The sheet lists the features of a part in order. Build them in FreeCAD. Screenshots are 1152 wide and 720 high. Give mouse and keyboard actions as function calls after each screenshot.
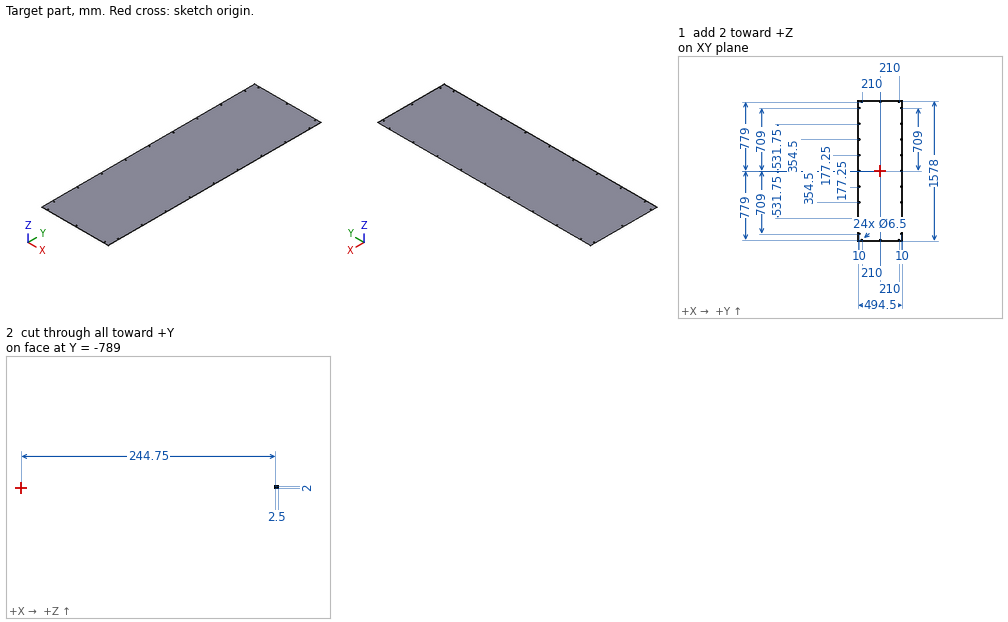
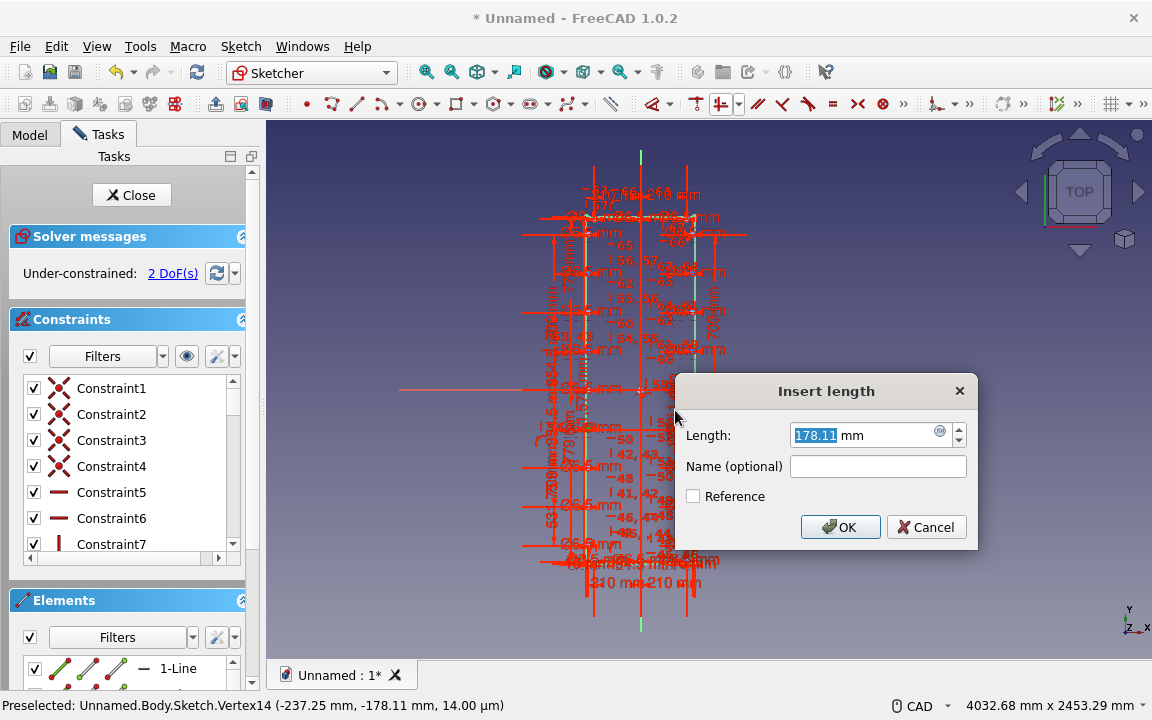
text(177.25)
key(Return)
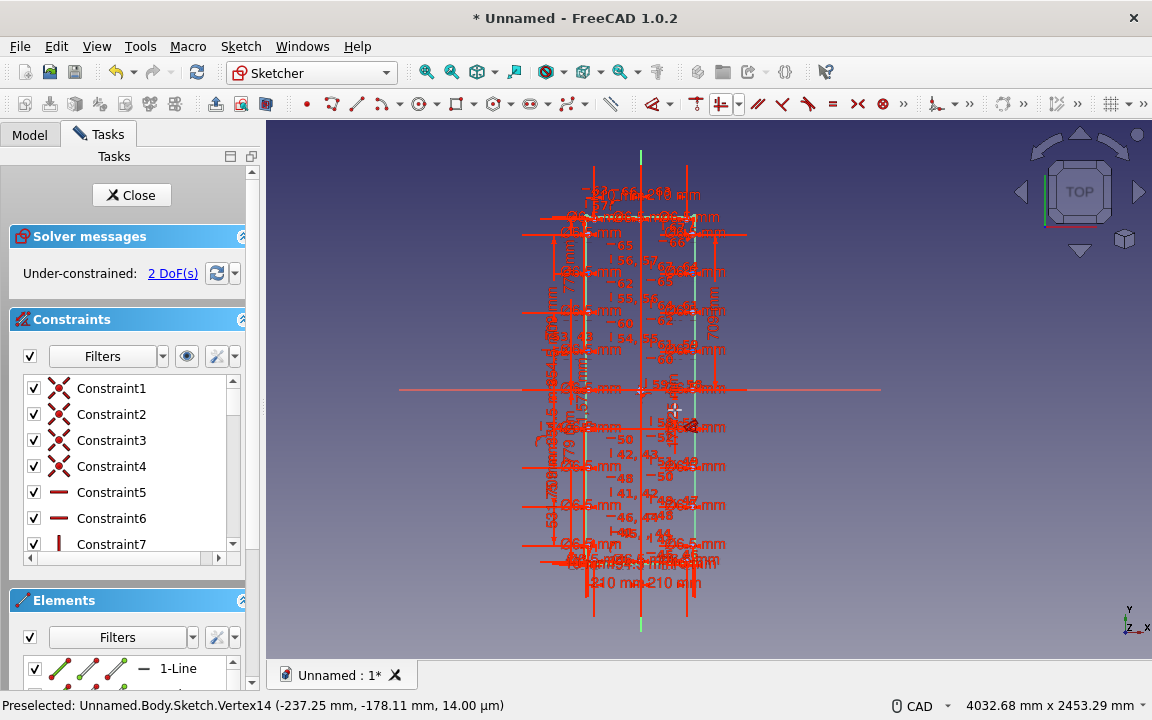
click(588, 352)
click(675, 371)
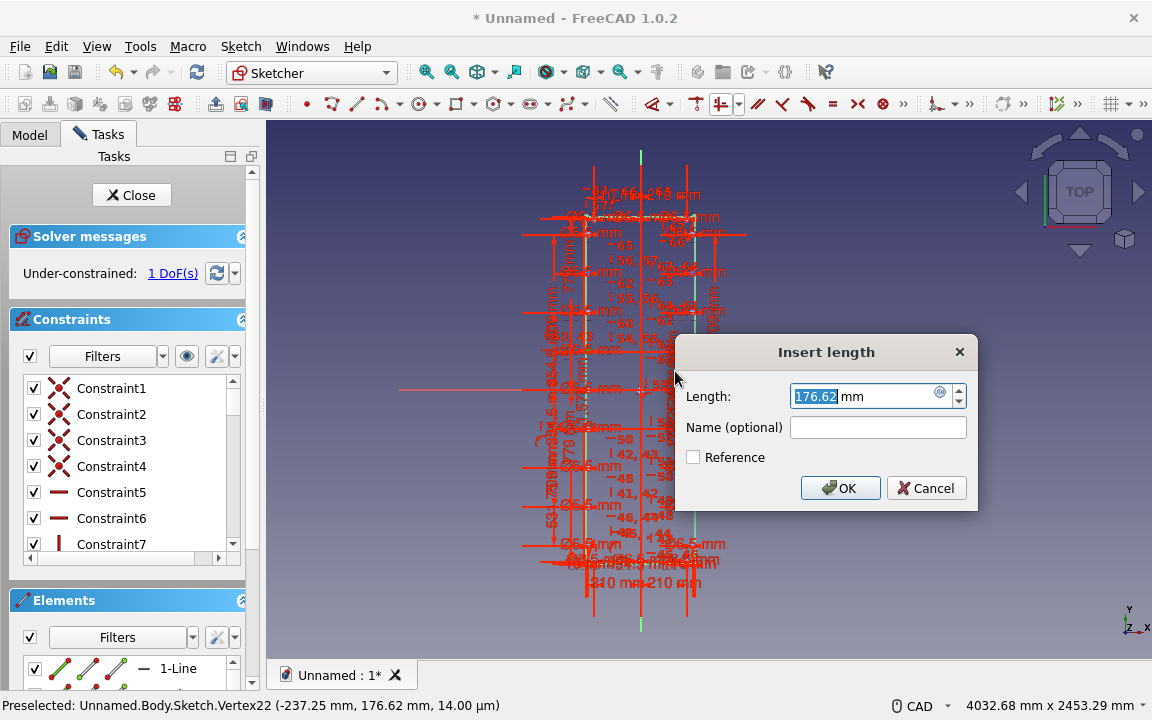
text(177.25)
key(Return)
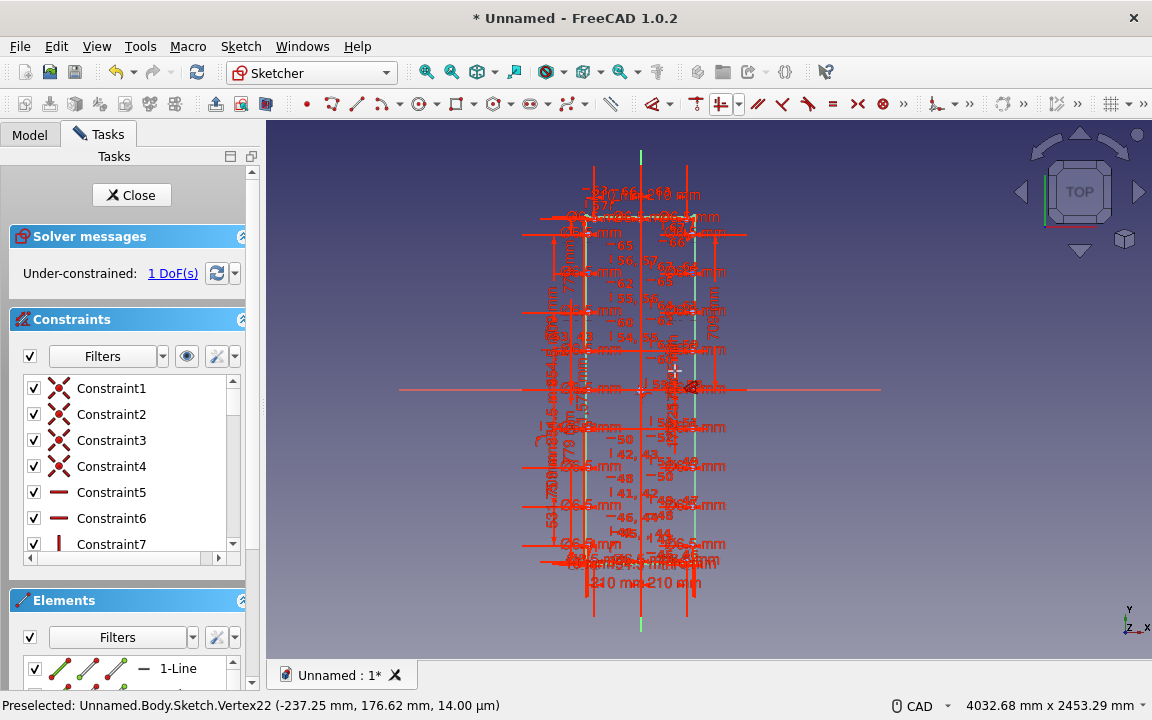
click(588, 274)
click(554, 291)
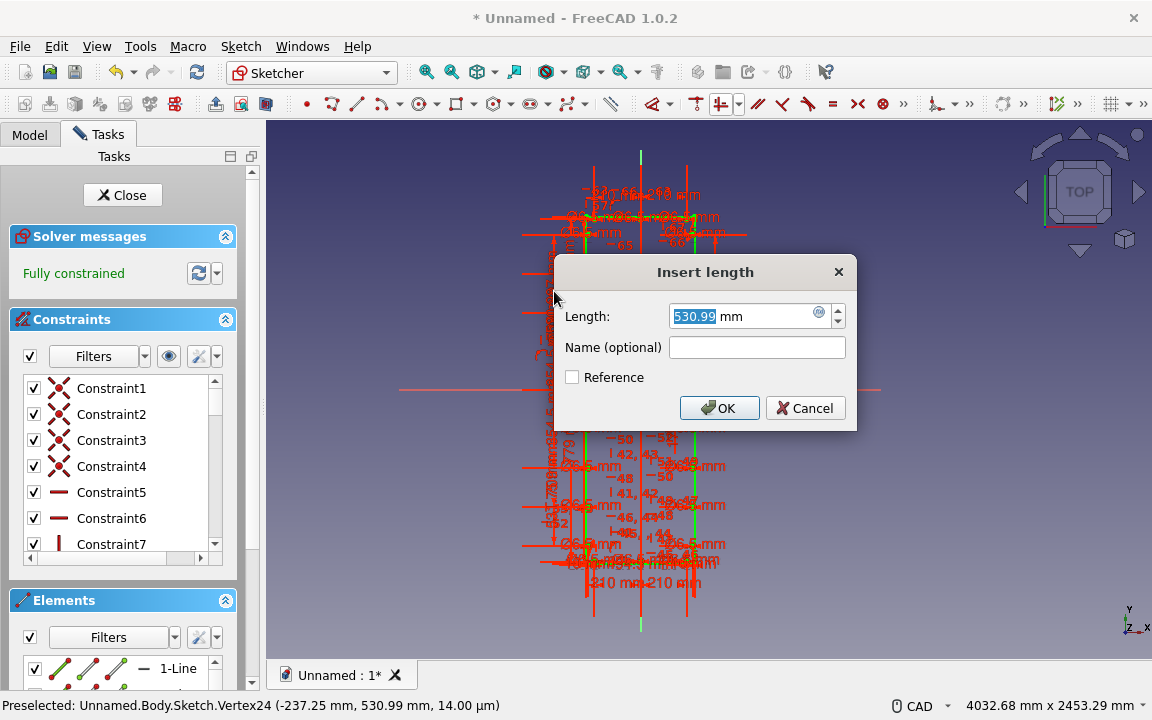
text(531.75)
key(Return)
key(Escape)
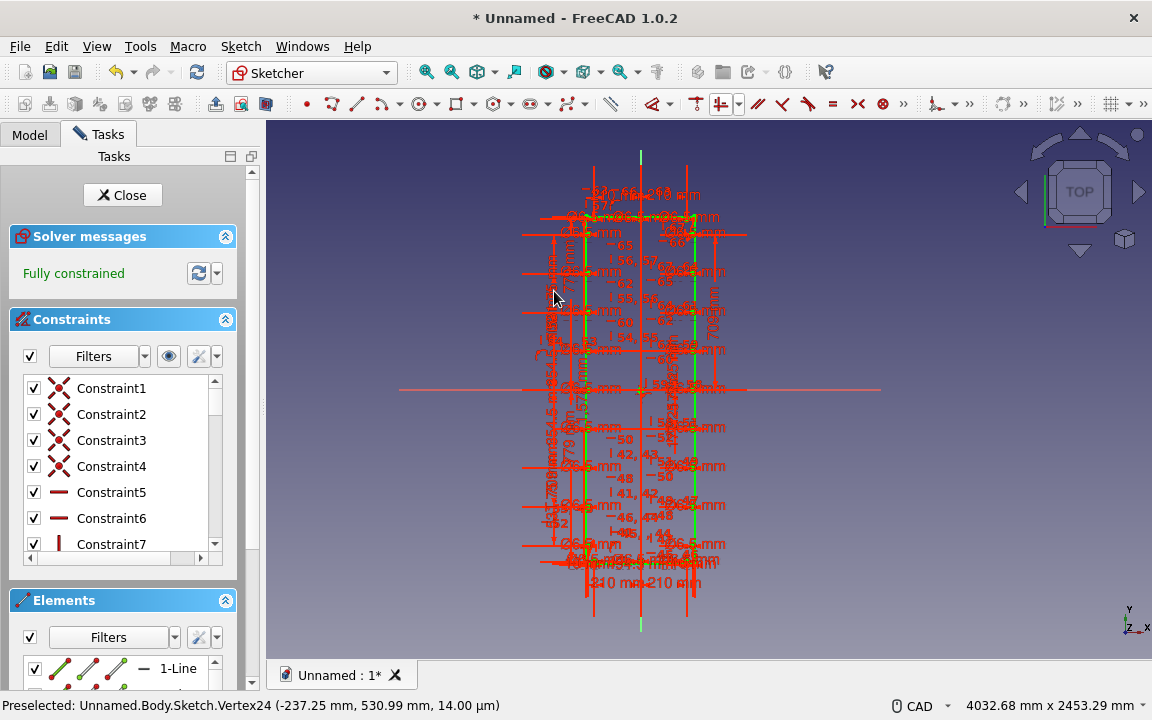
click(123, 195)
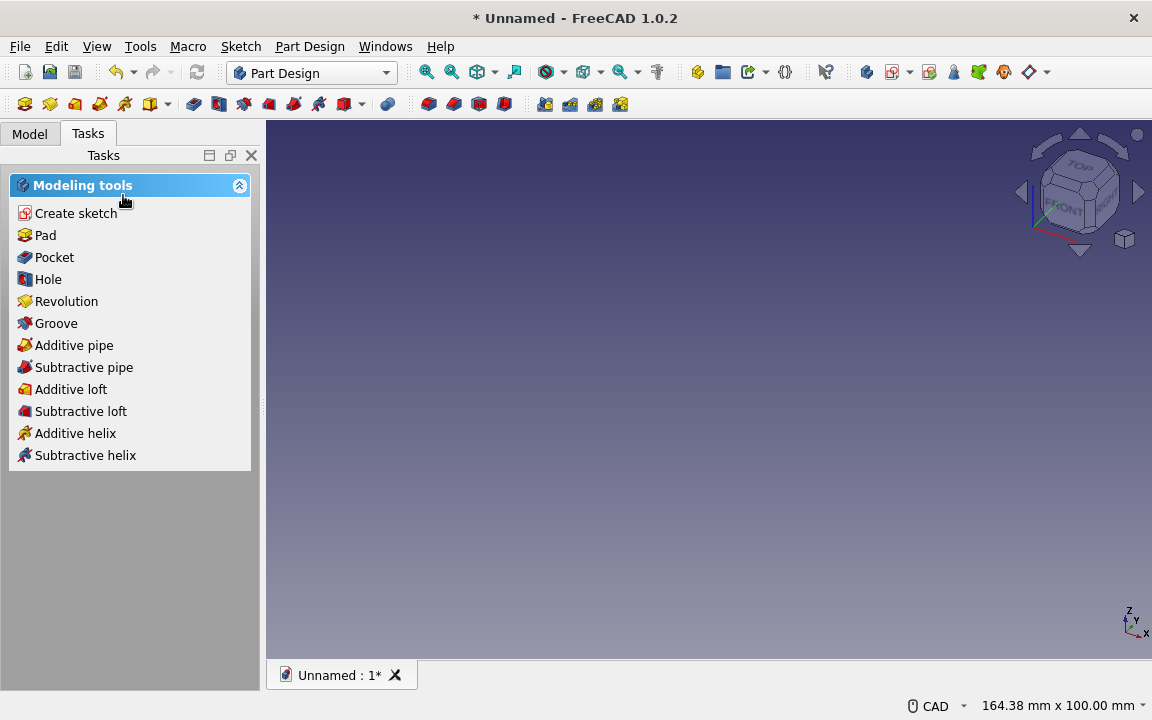
click(25, 104)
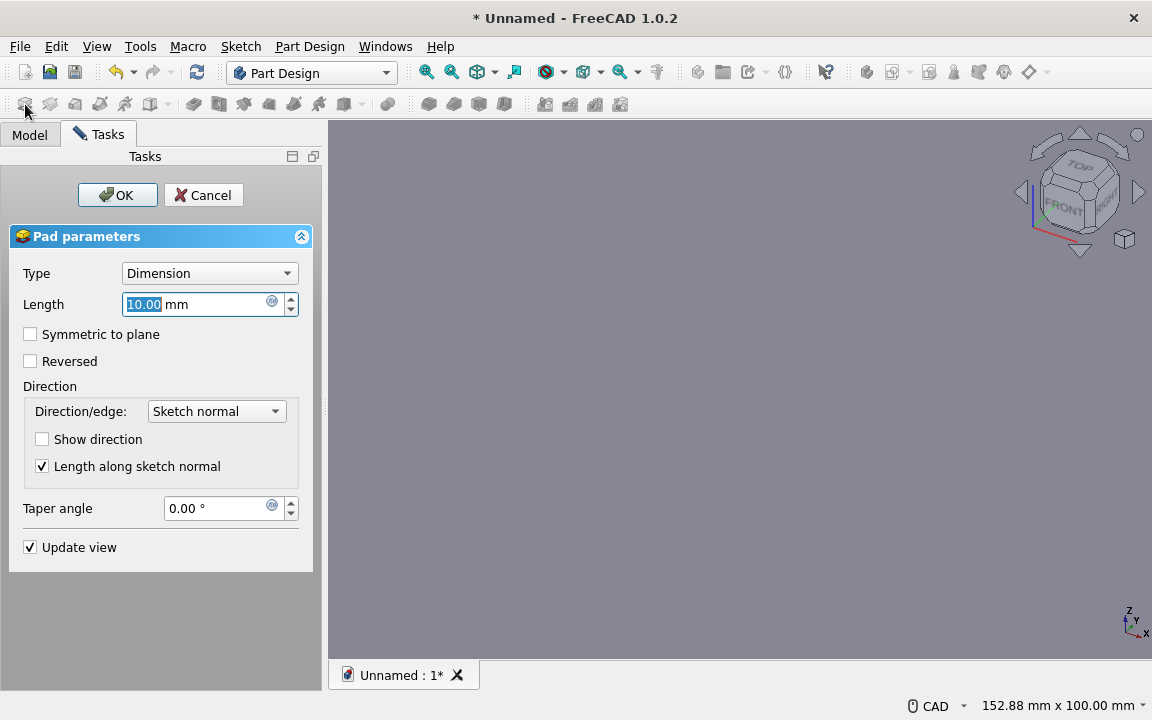
text(2)
key(Tab)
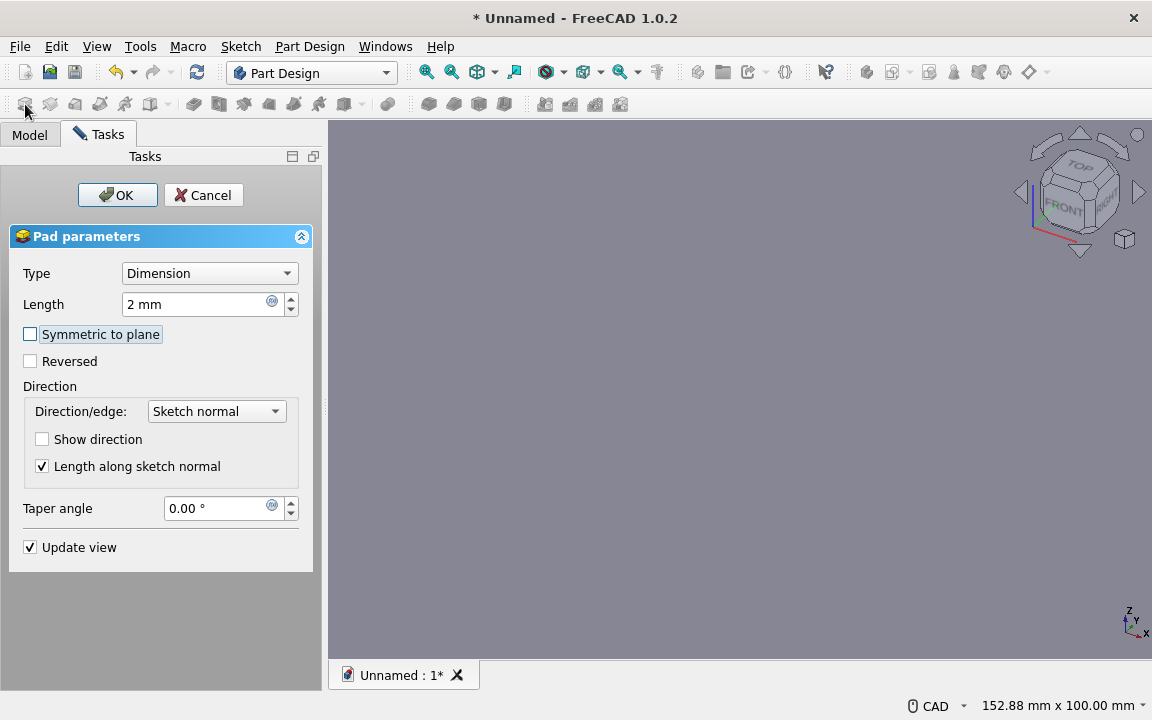
click(118, 195)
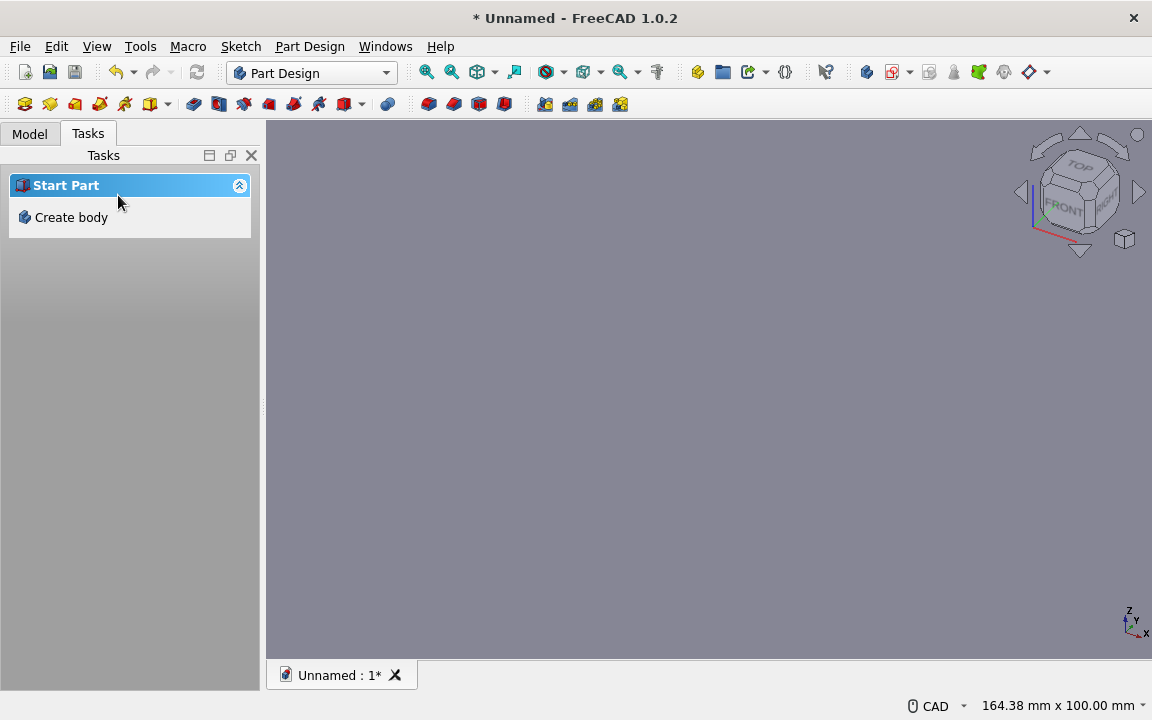
click(427, 72)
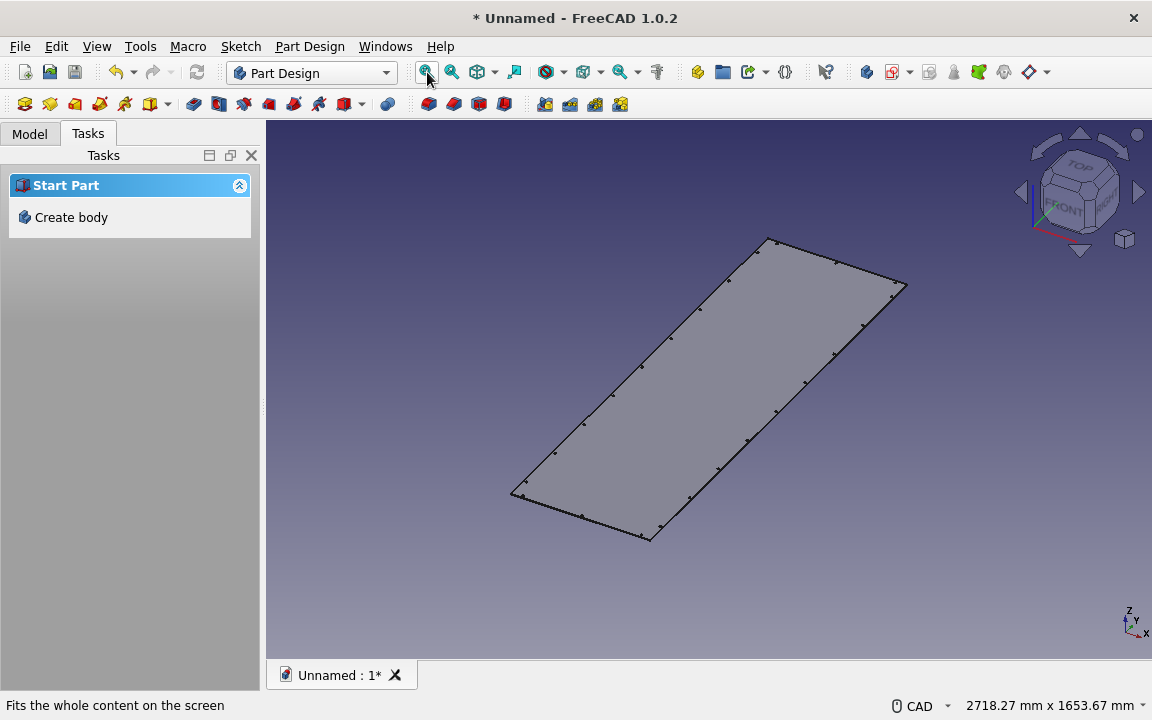
scroll(640, 536, up, 15)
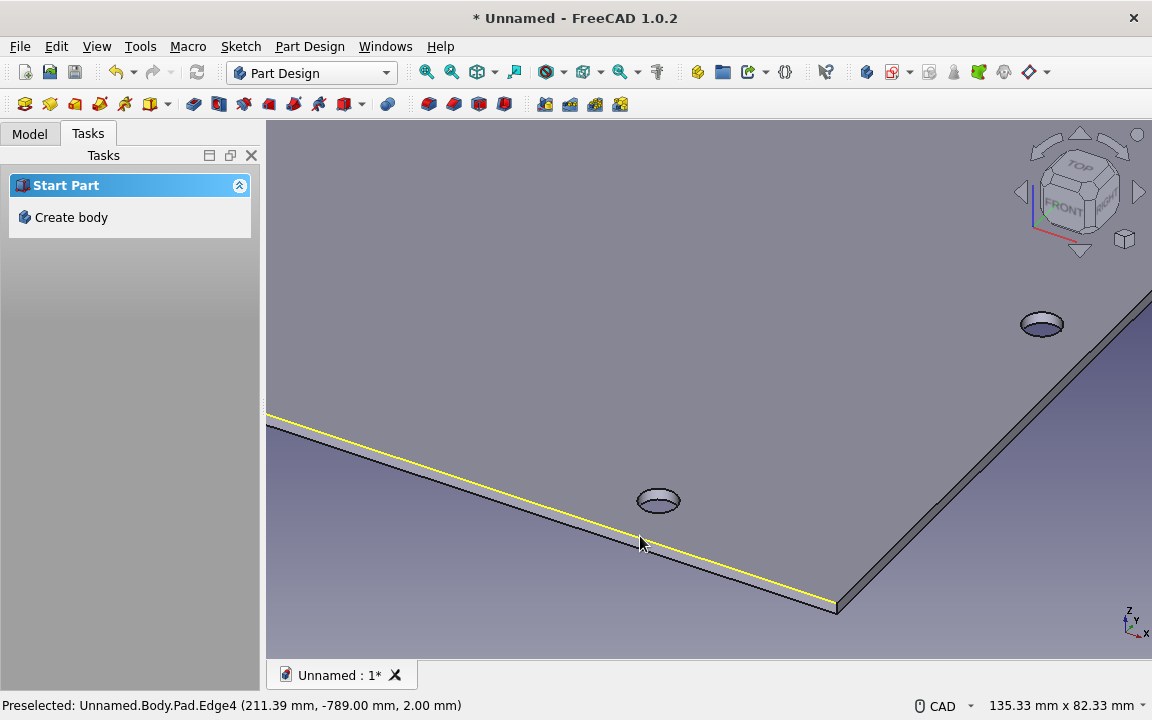
scroll(637, 541, up, 4)